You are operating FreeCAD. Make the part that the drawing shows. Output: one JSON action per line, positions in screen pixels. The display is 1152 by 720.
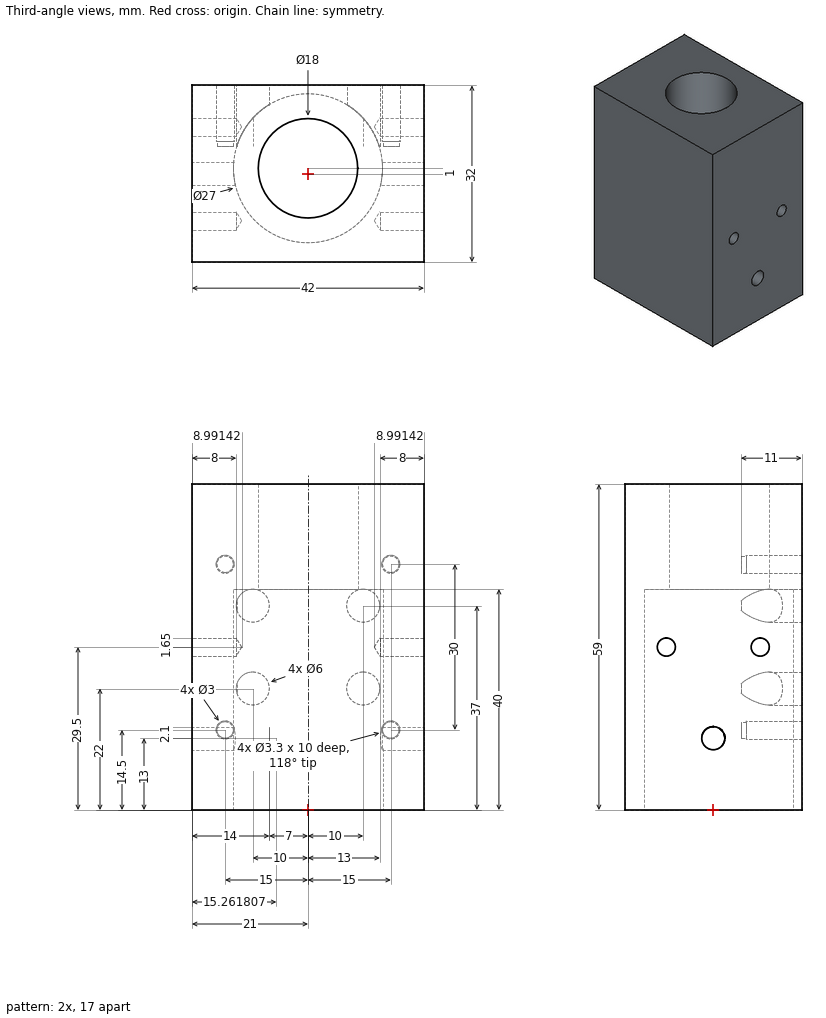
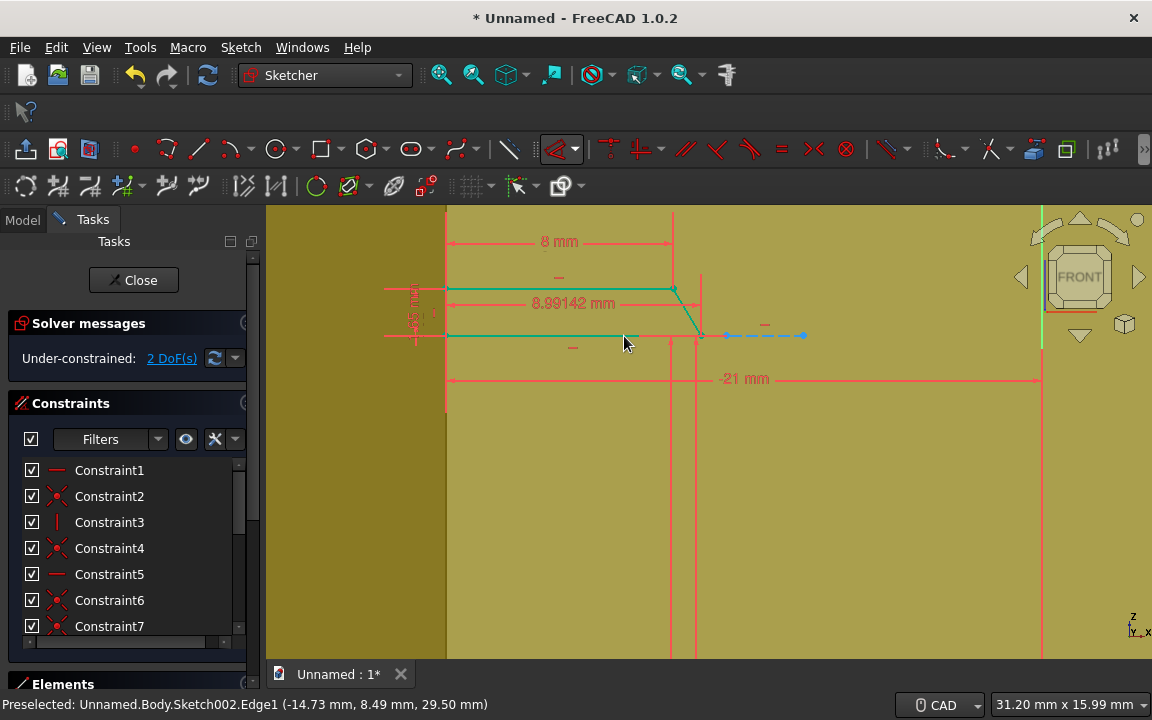
{"action": "left_click", "coordinate": [134, 280]}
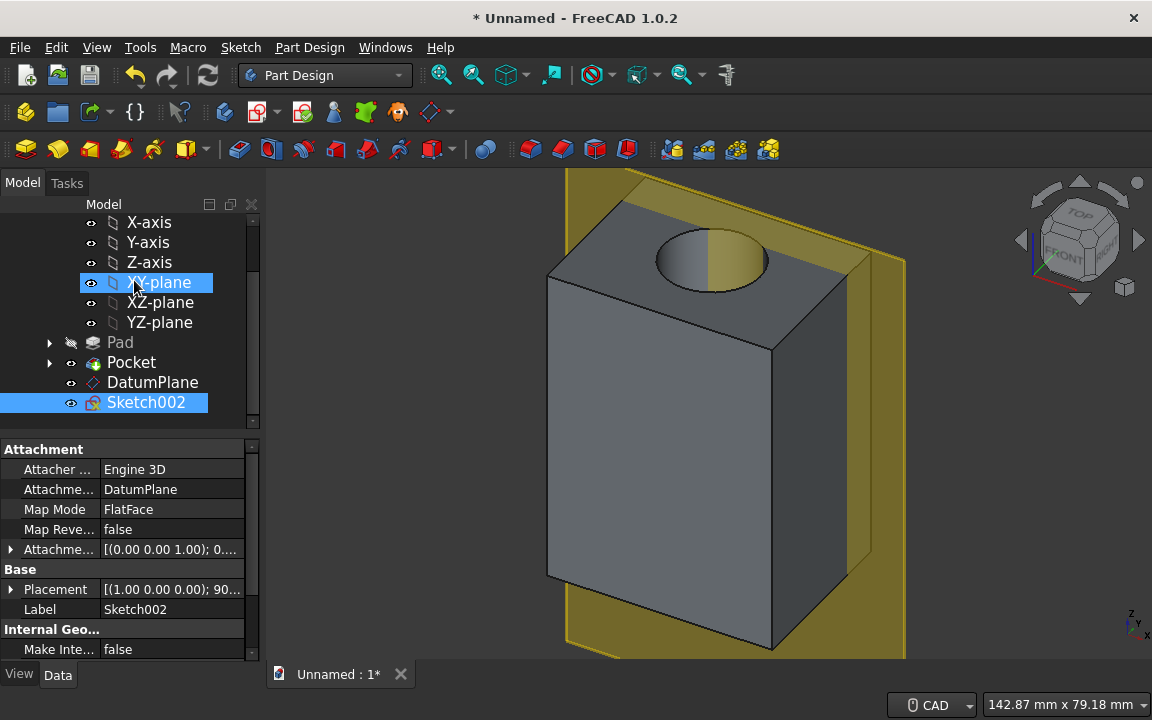
{"action": "left_click", "coordinate": [304, 150]}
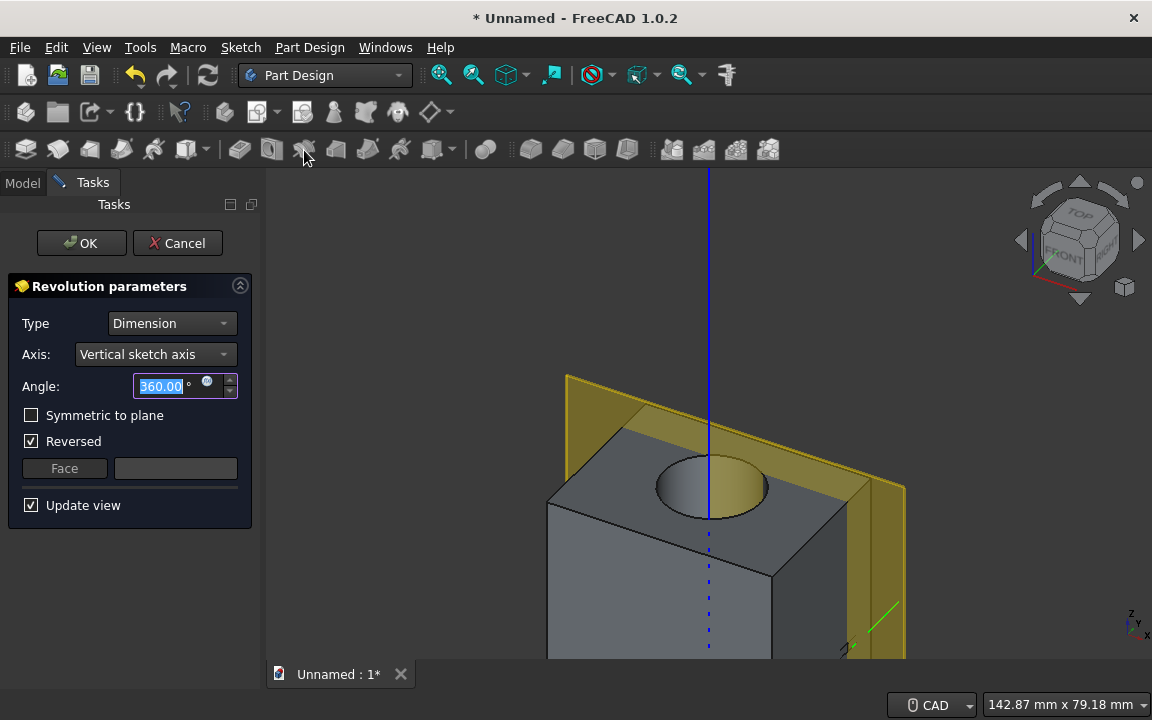
{"action": "left_click", "coordinate": [156, 354]}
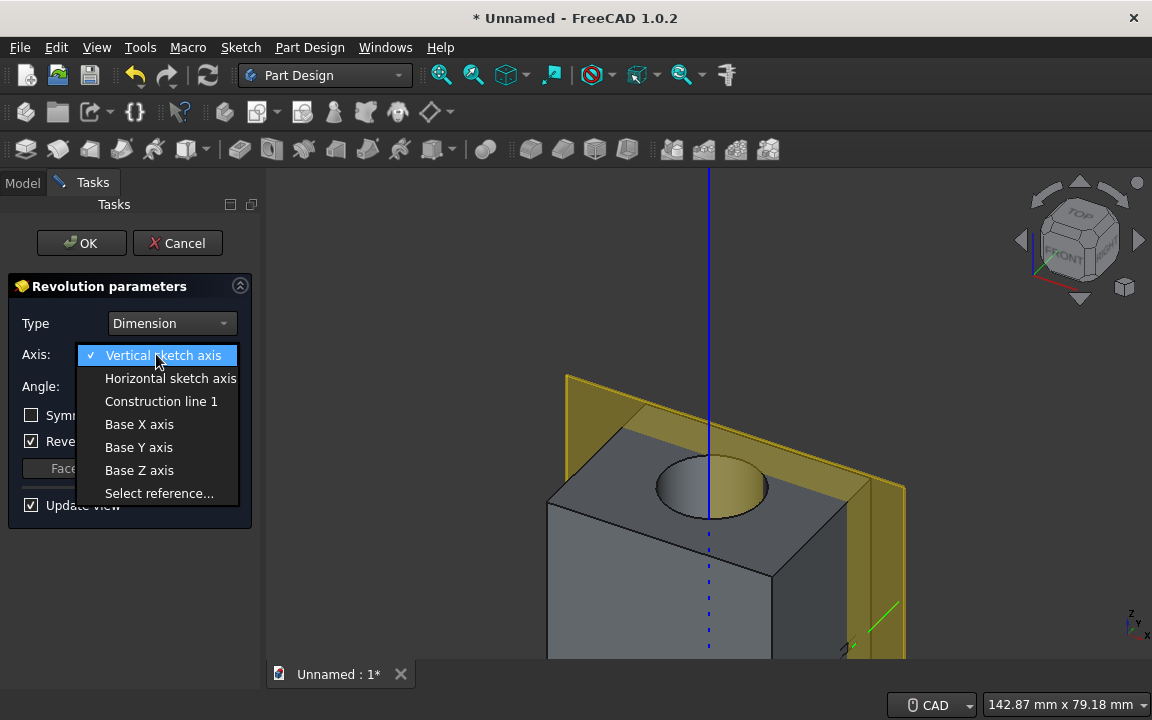
{"action": "left_click", "coordinate": [156, 402]}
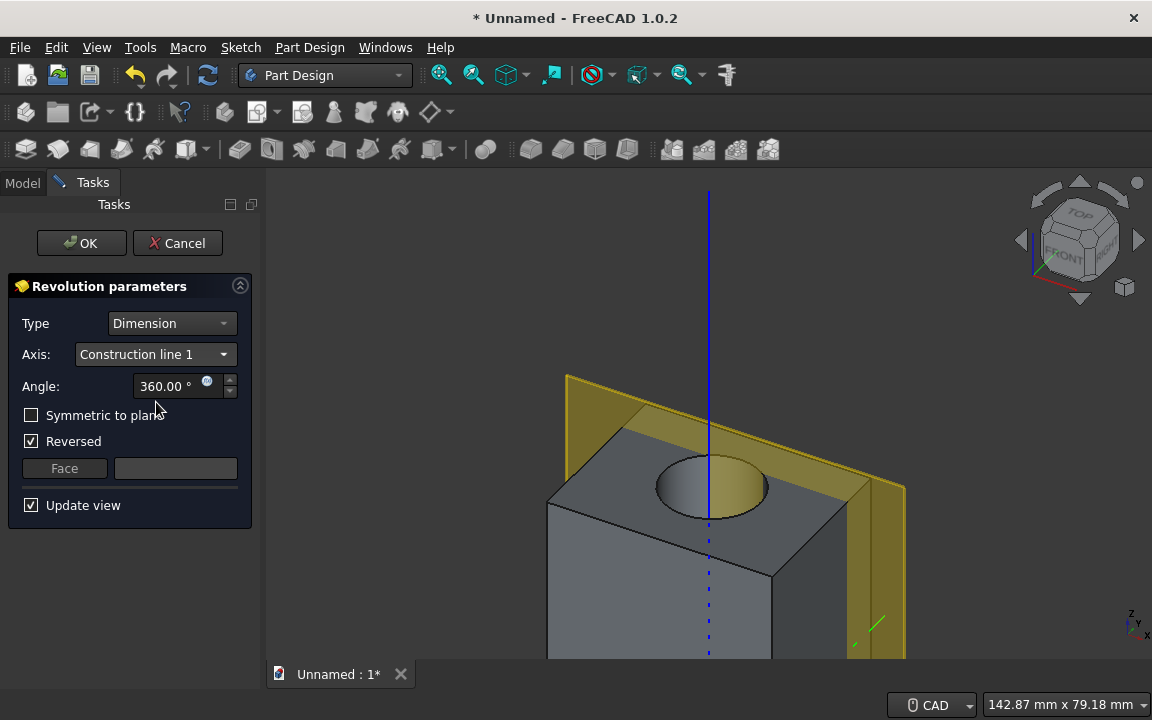
{"action": "left_click", "coordinate": [82, 243]}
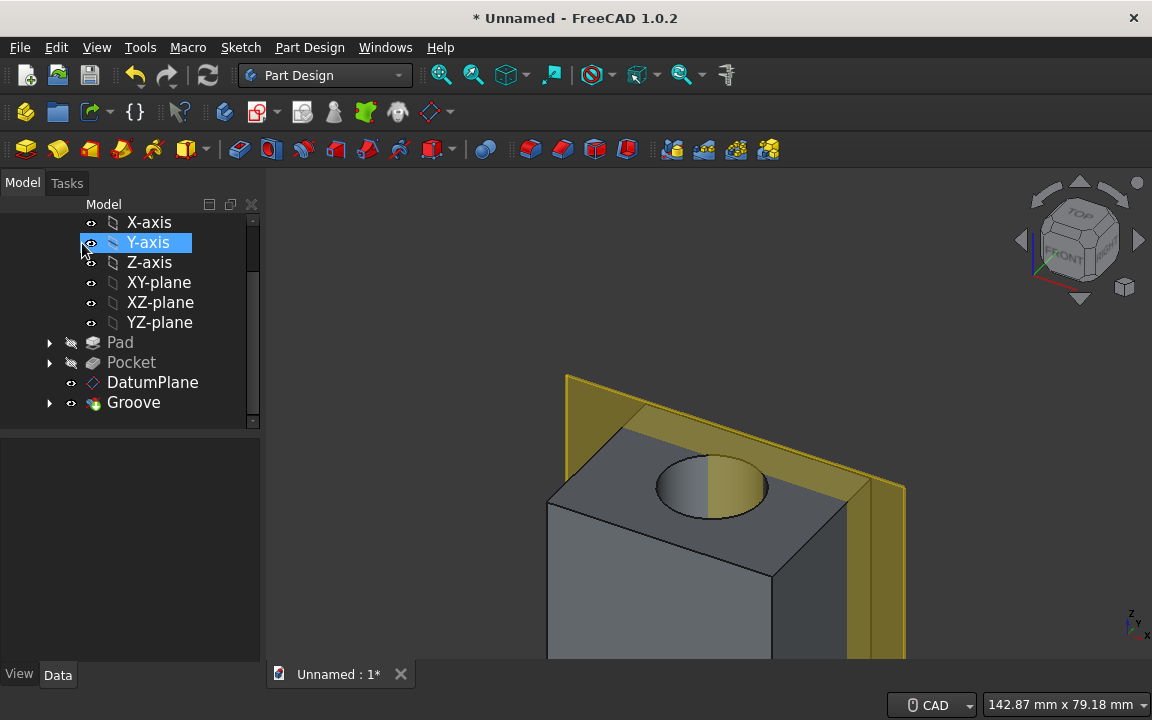
{"action": "left_click", "coordinate": [116, 383]}
{"action": "key", "text": "space"}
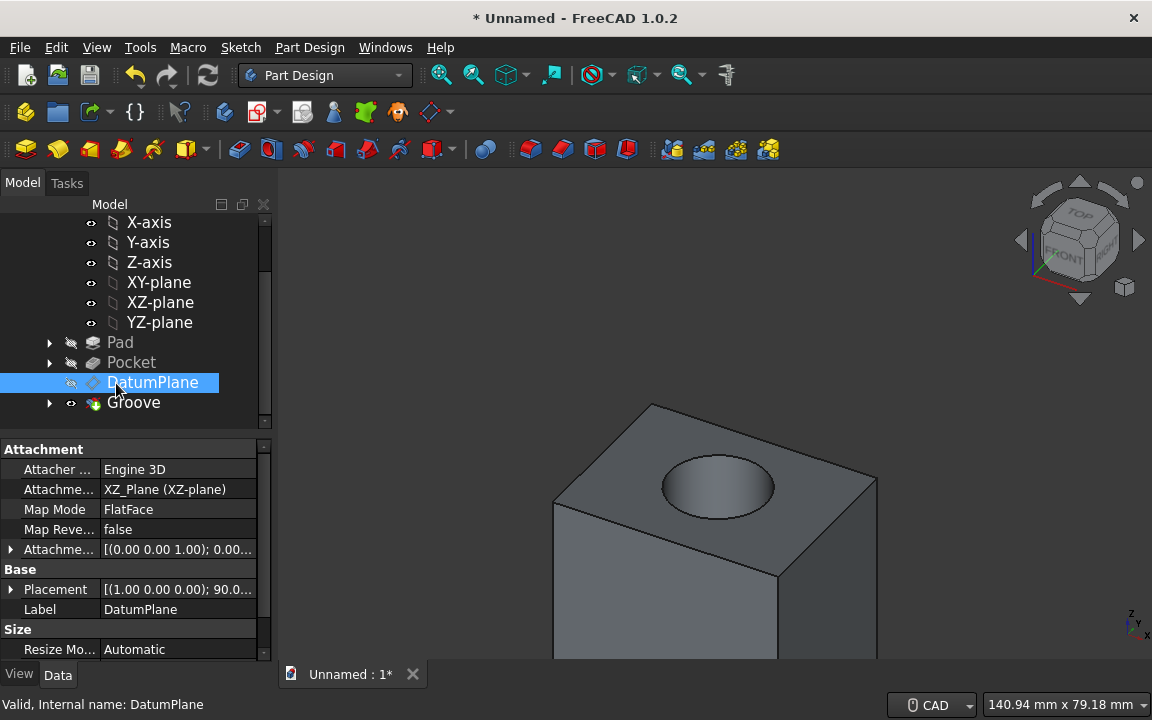
{"action": "key", "text": "v f"}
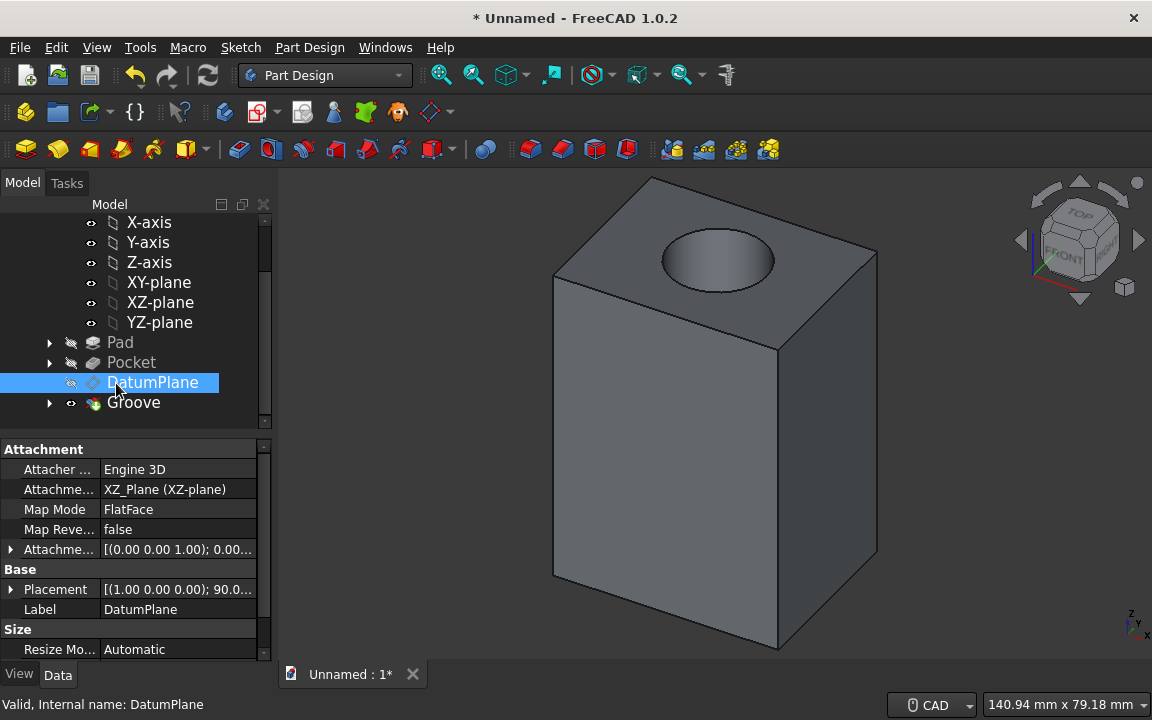
{"action": "left_click", "coordinate": [116, 403]}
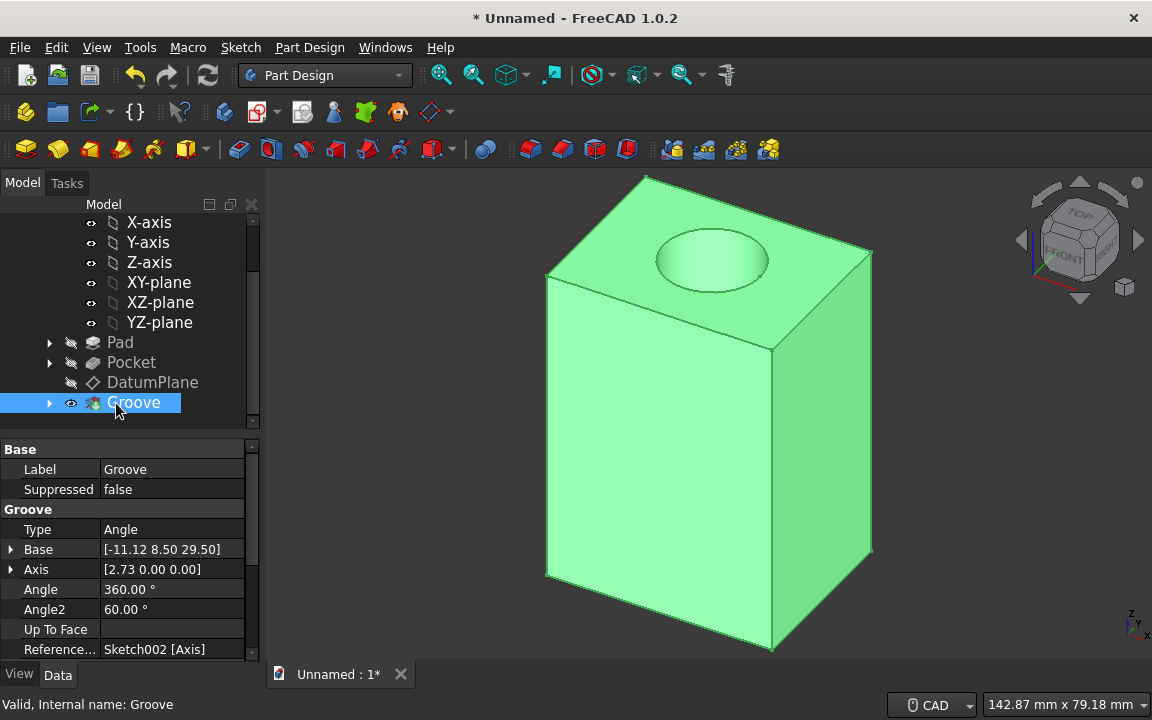
{"action": "left_click", "coordinate": [704, 150]}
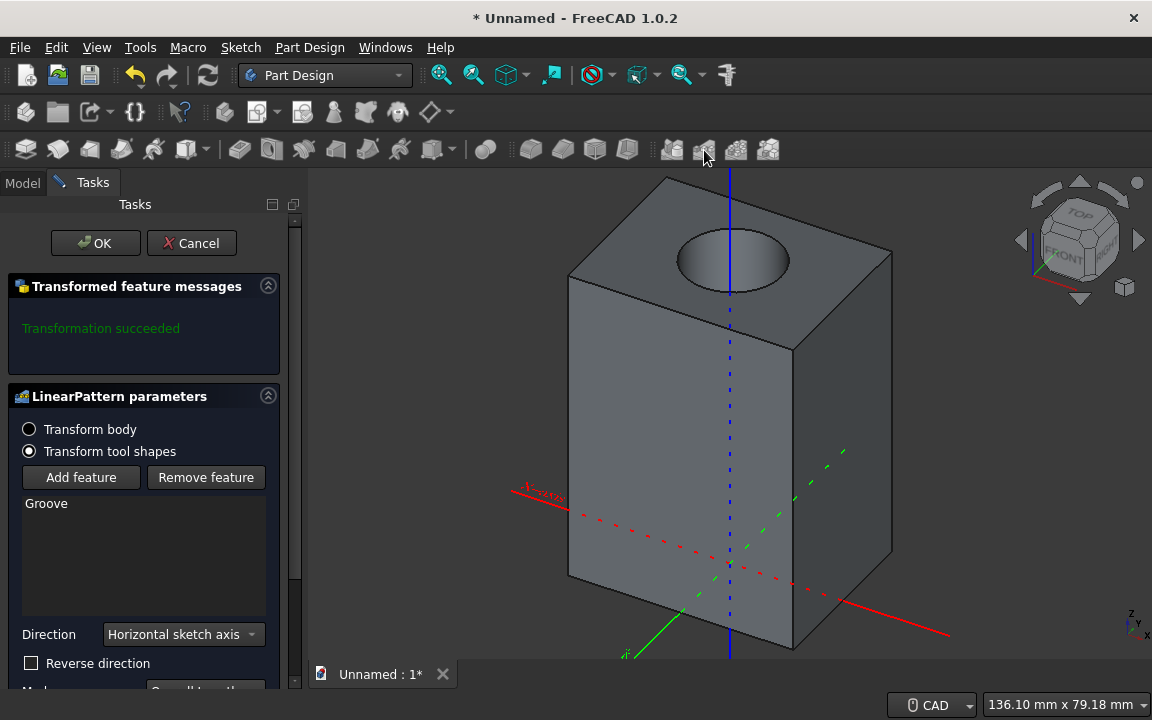
{"action": "left_click", "coordinate": [184, 634]}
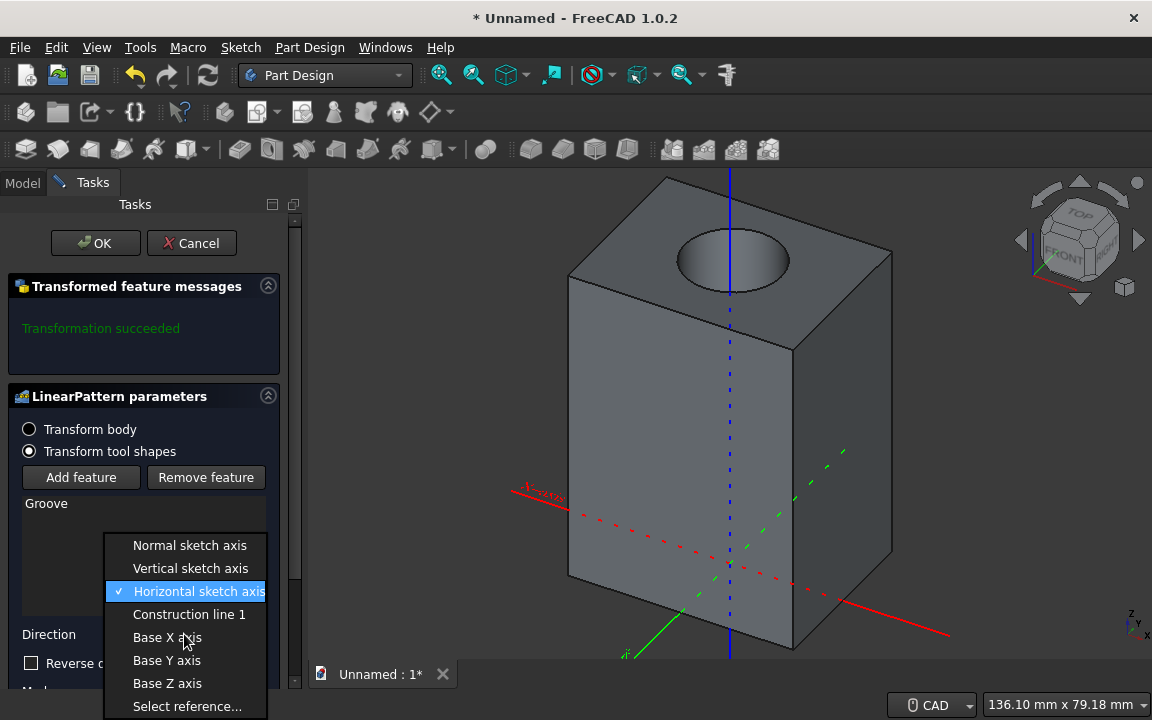
{"action": "left_click", "coordinate": [184, 660]}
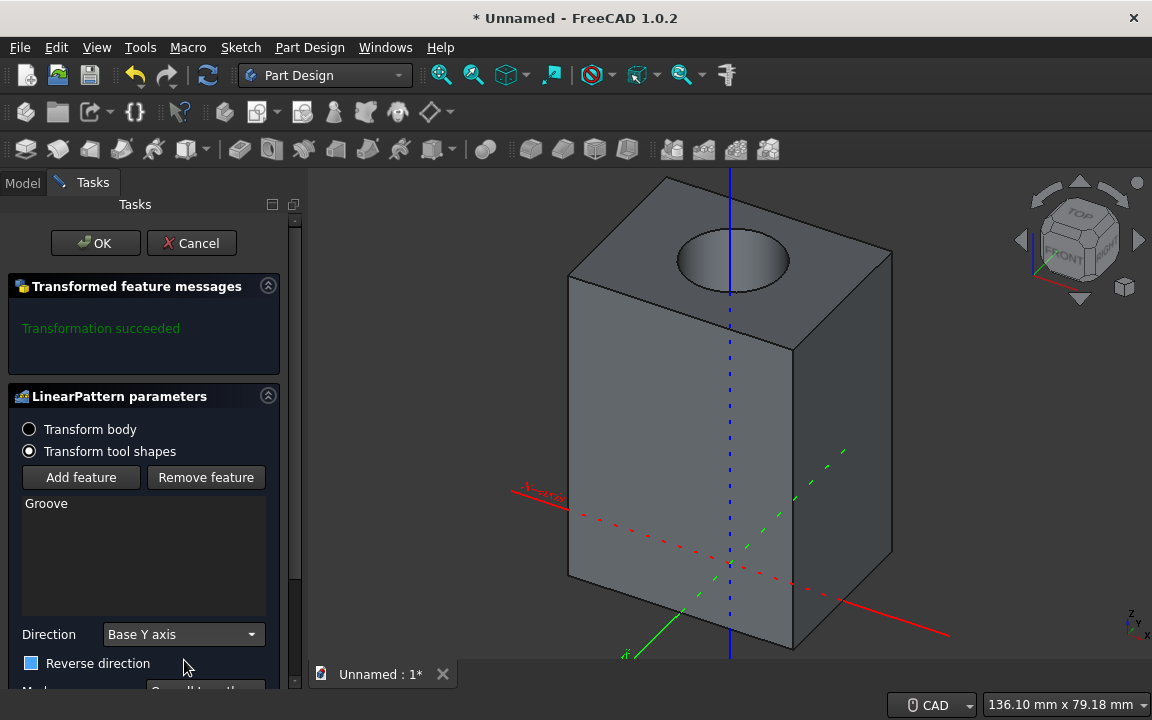
{"action": "scroll", "coordinate": [295, 451], "scroll_direction": "down", "scroll_amount": 2}